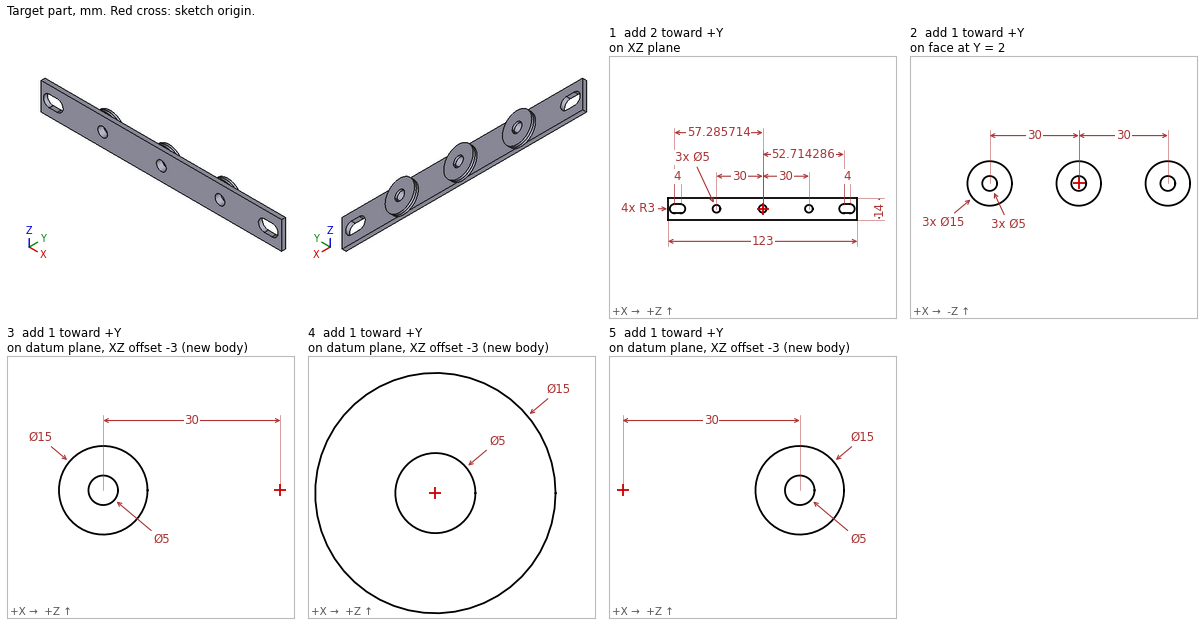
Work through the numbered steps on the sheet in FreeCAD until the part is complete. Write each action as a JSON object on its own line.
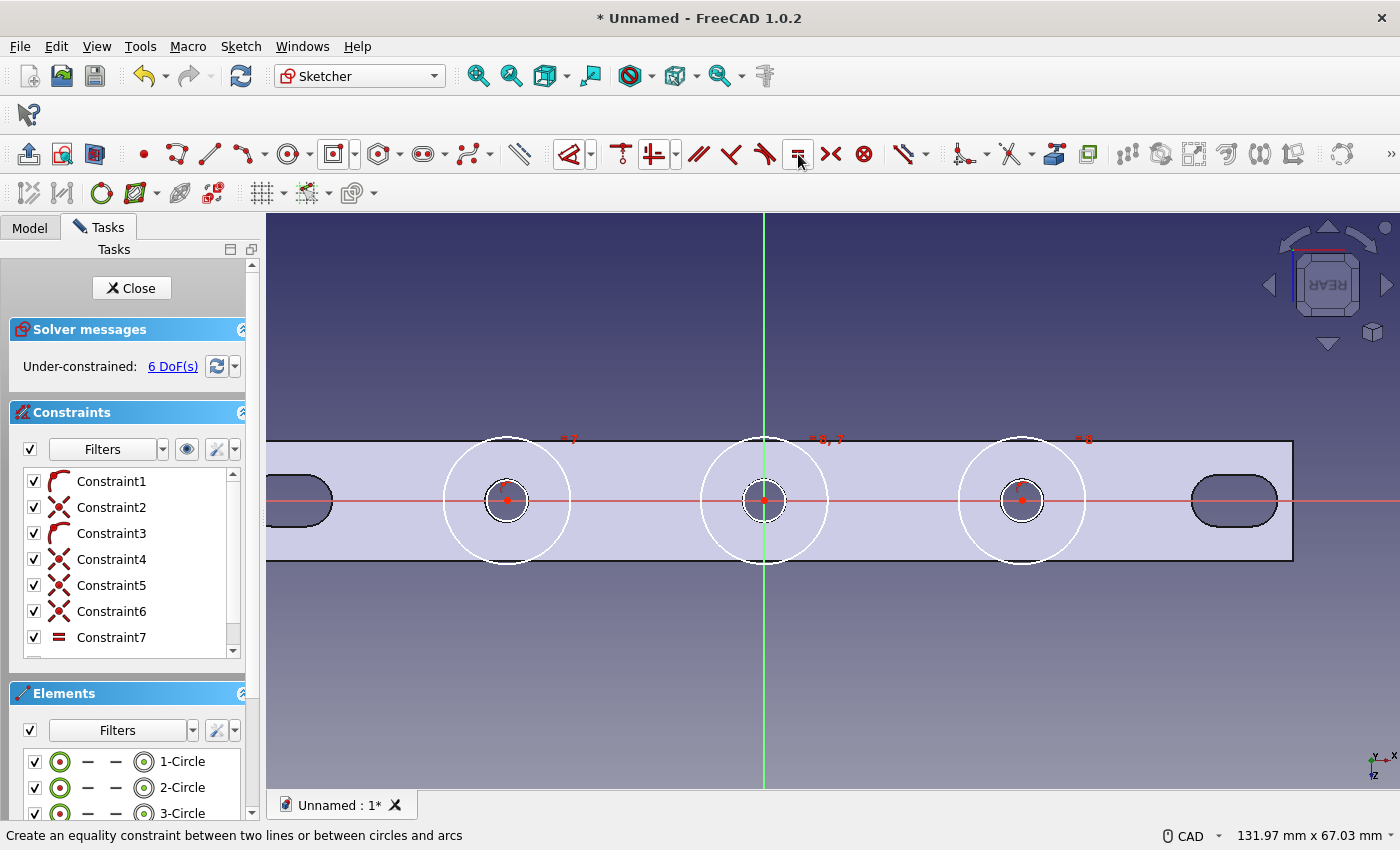
{"action": "left_click", "coordinate": [521, 486]}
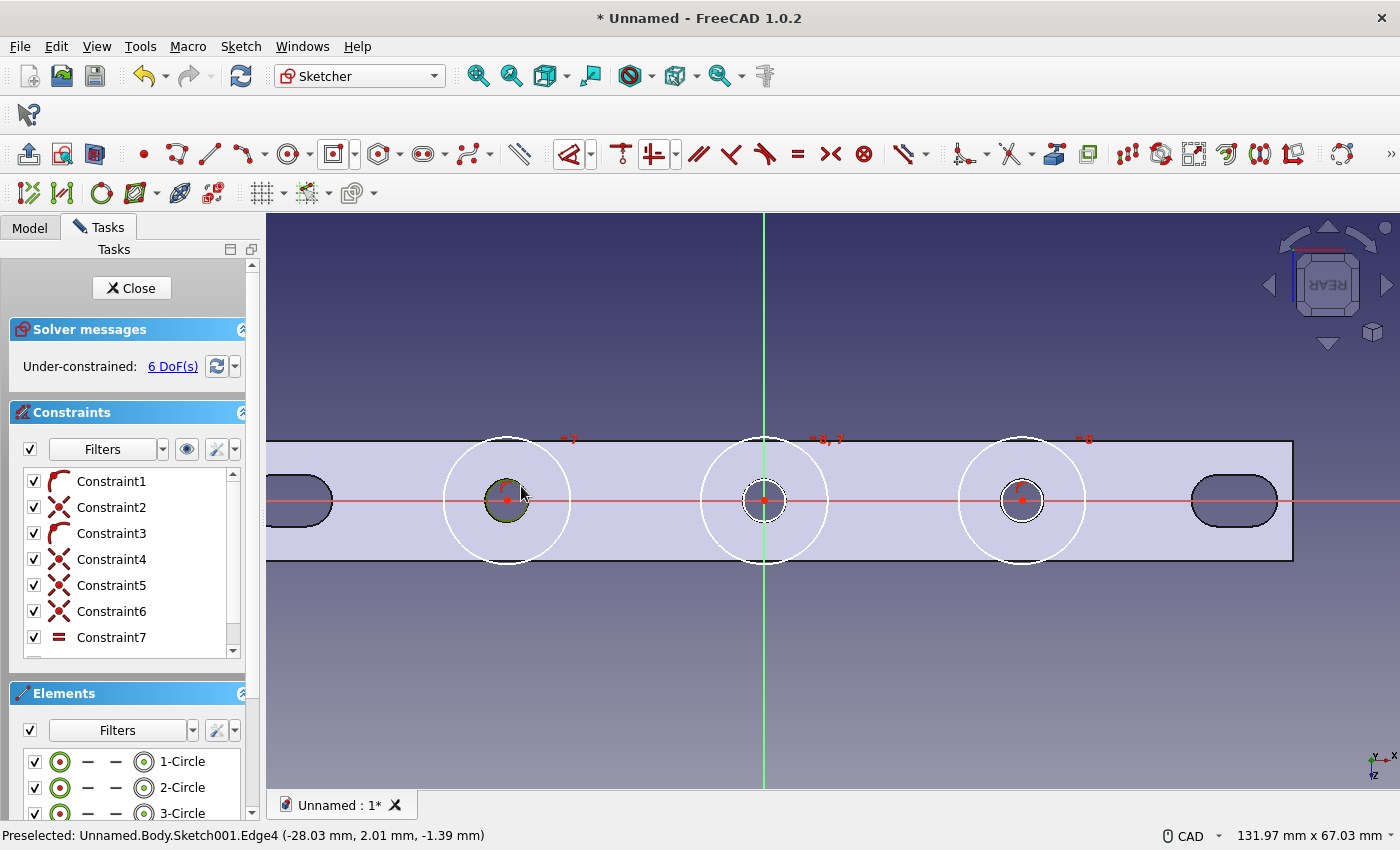
{"action": "left_click", "coordinate": [779, 486]}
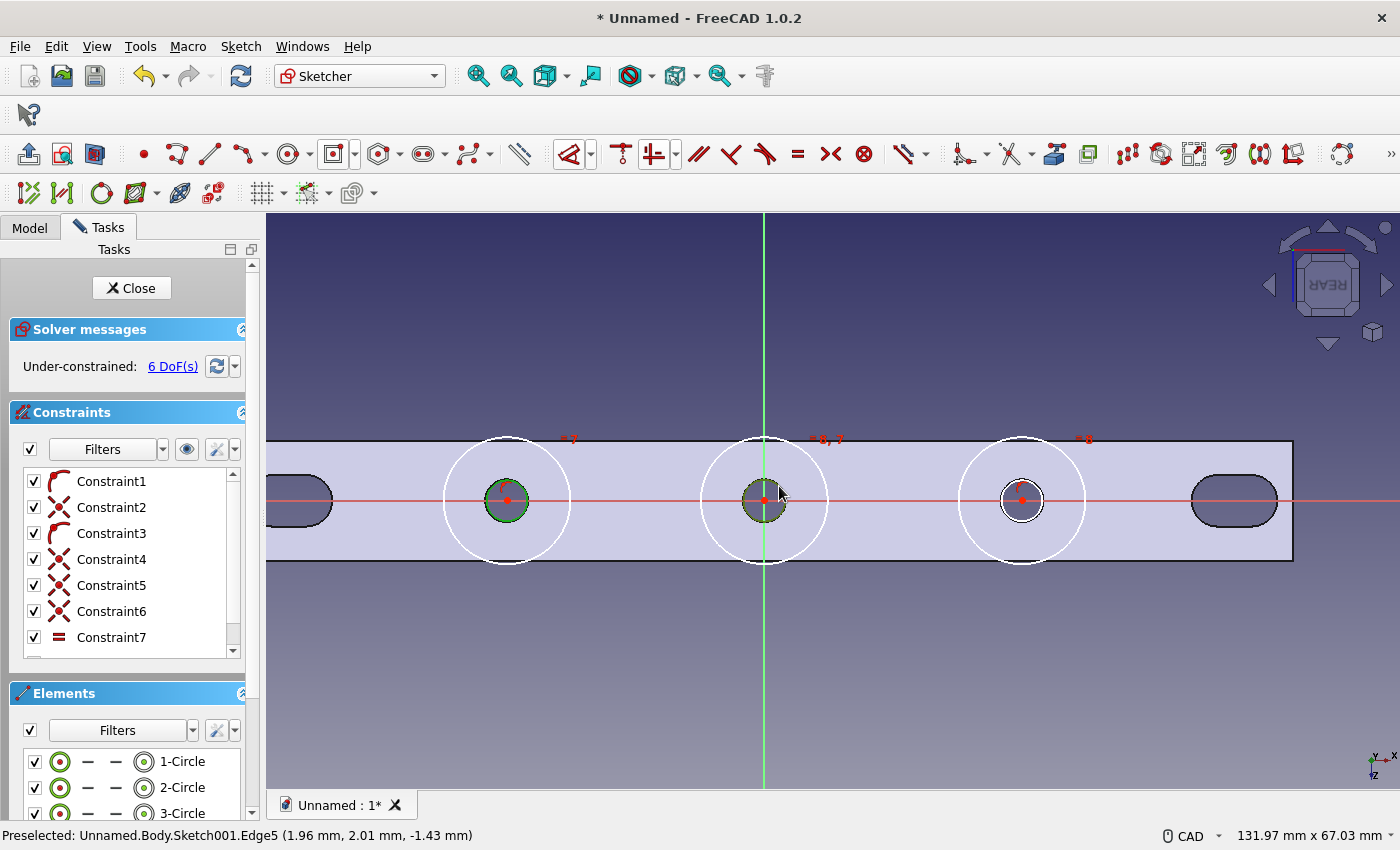
{"action": "left_click", "coordinate": [1036, 486]}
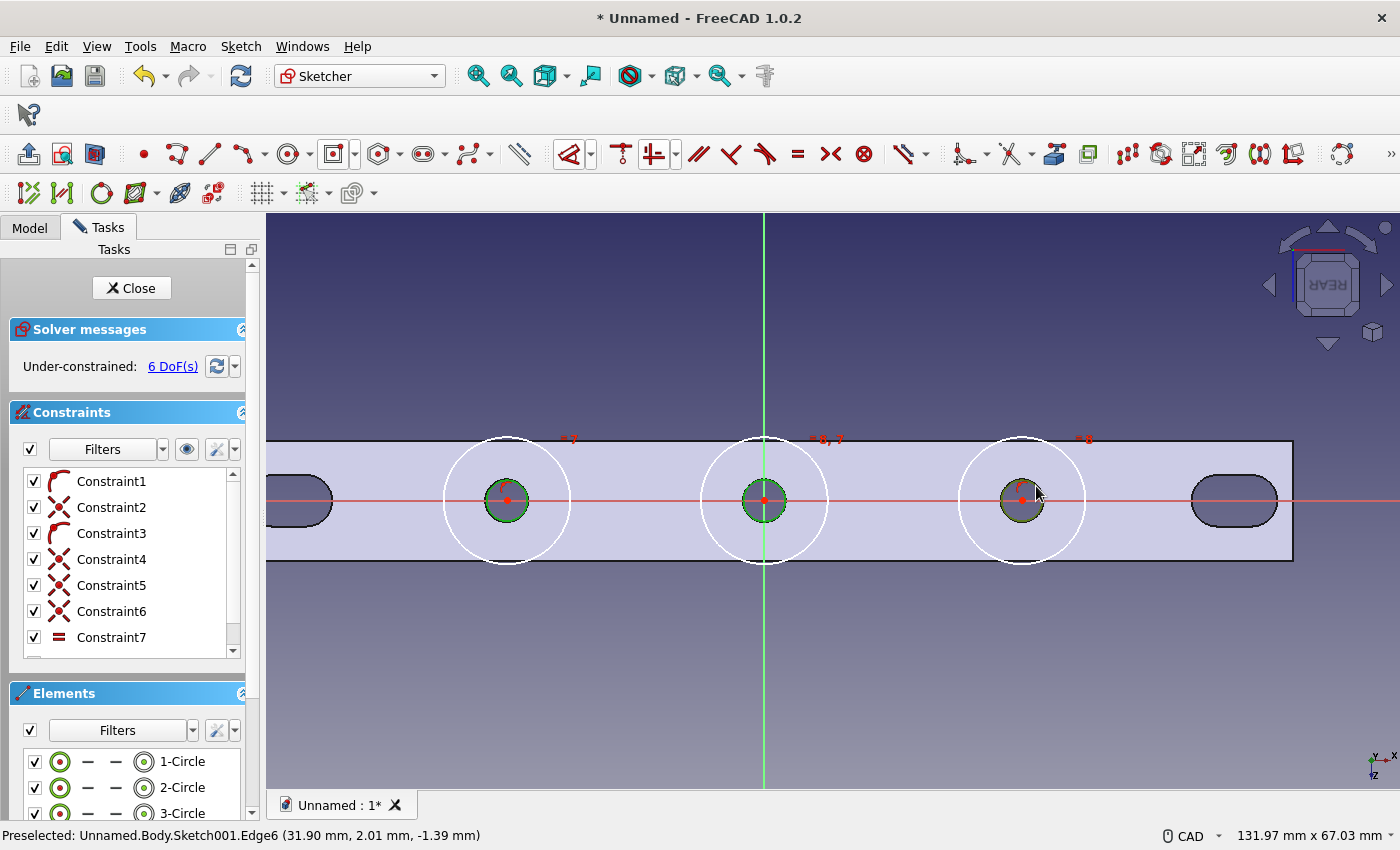
{"action": "left_click", "coordinate": [798, 154]}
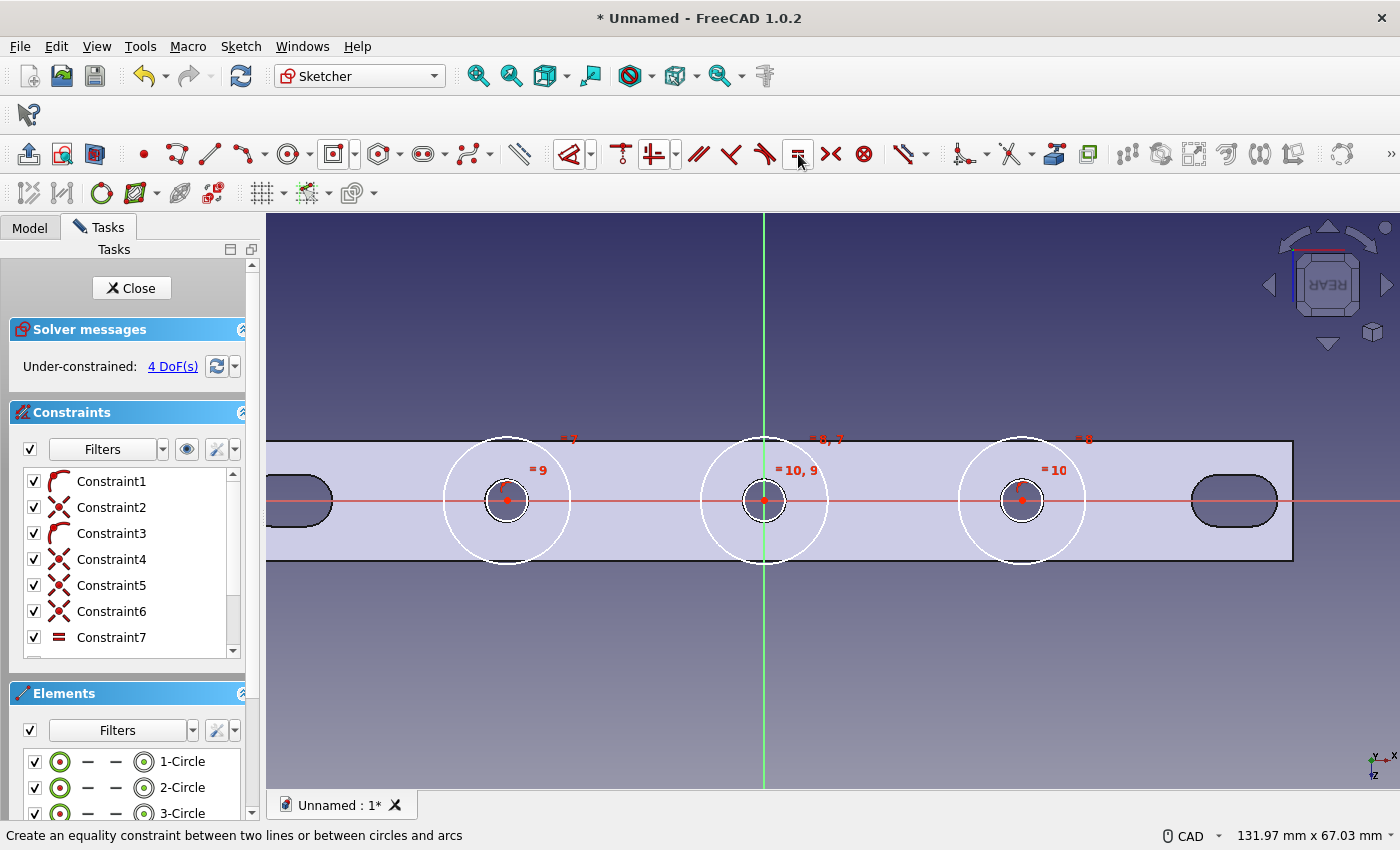
{"action": "left_click", "coordinate": [552, 456]}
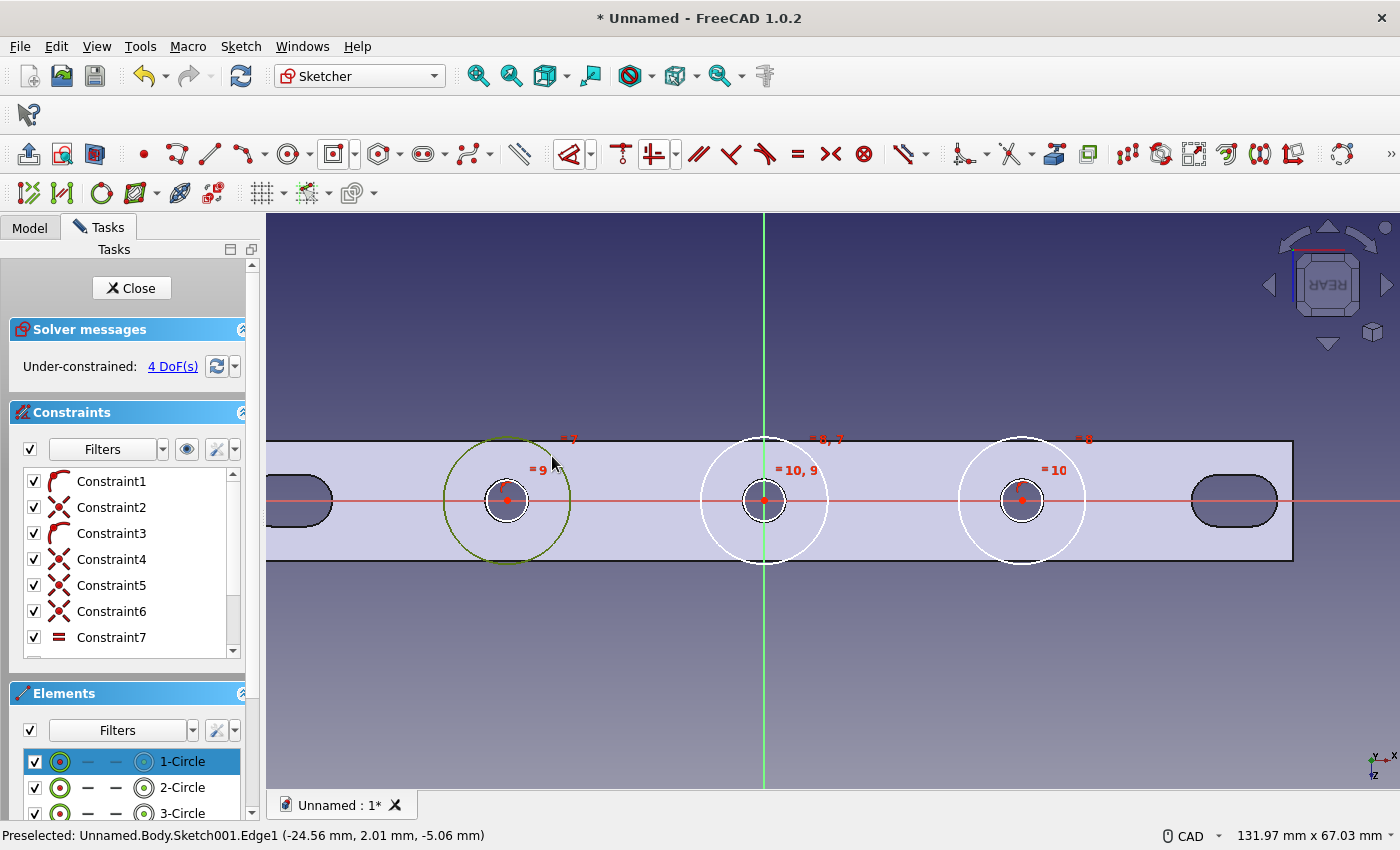
{"action": "key", "text": "k o"}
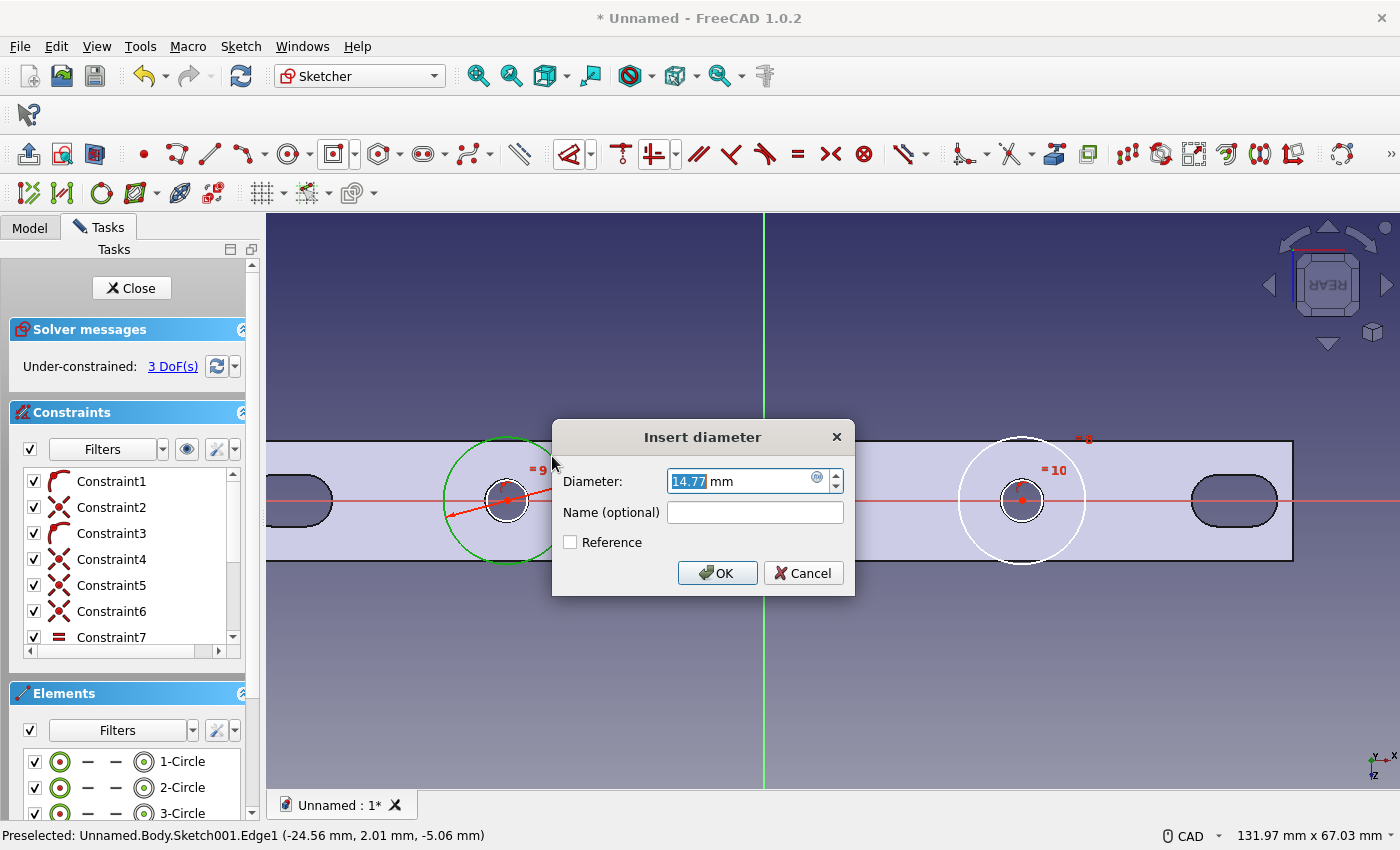
{"action": "type", "text": "15"}
{"action": "key", "text": "Return"}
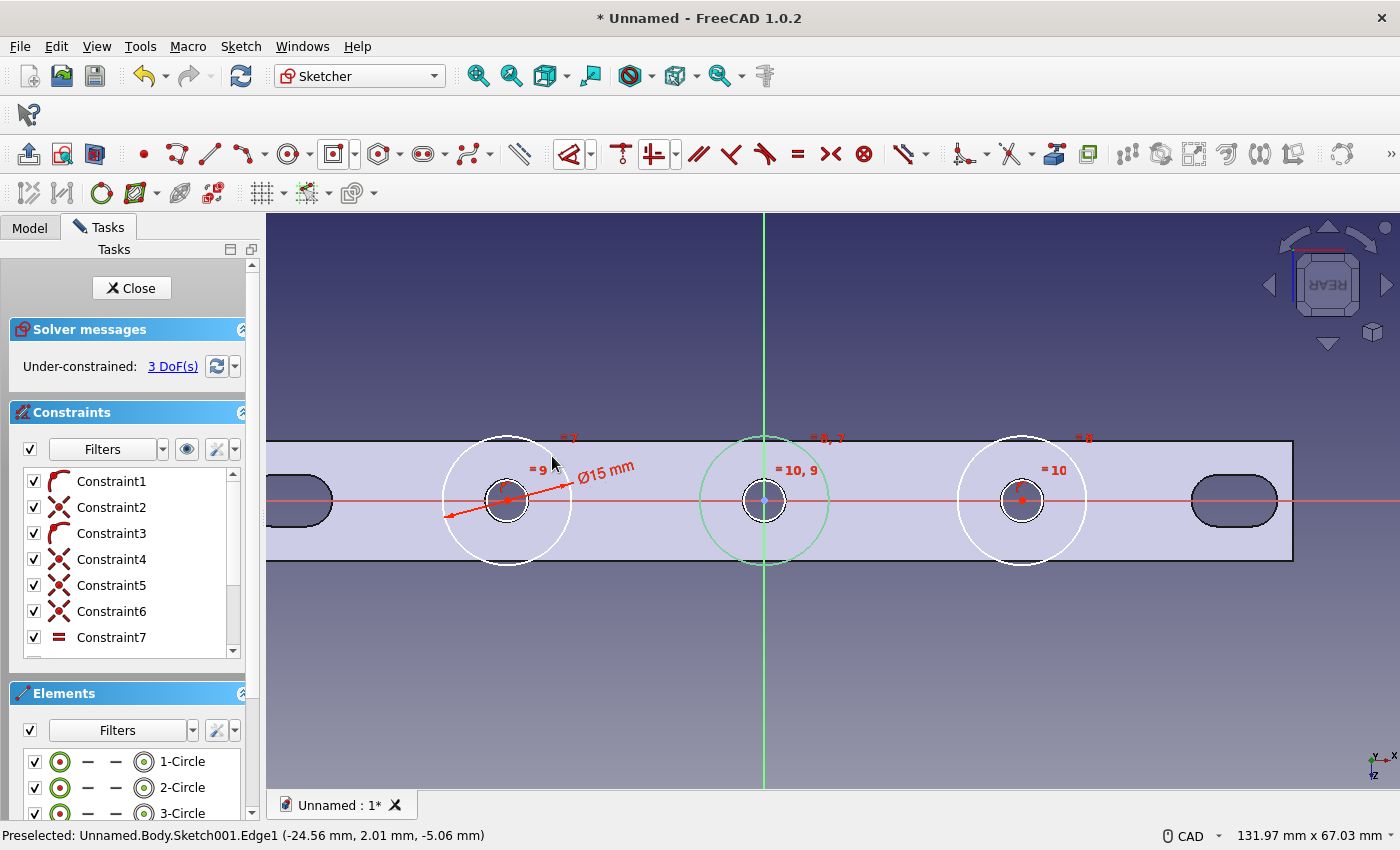
{"action": "left_click", "coordinate": [521, 486]}